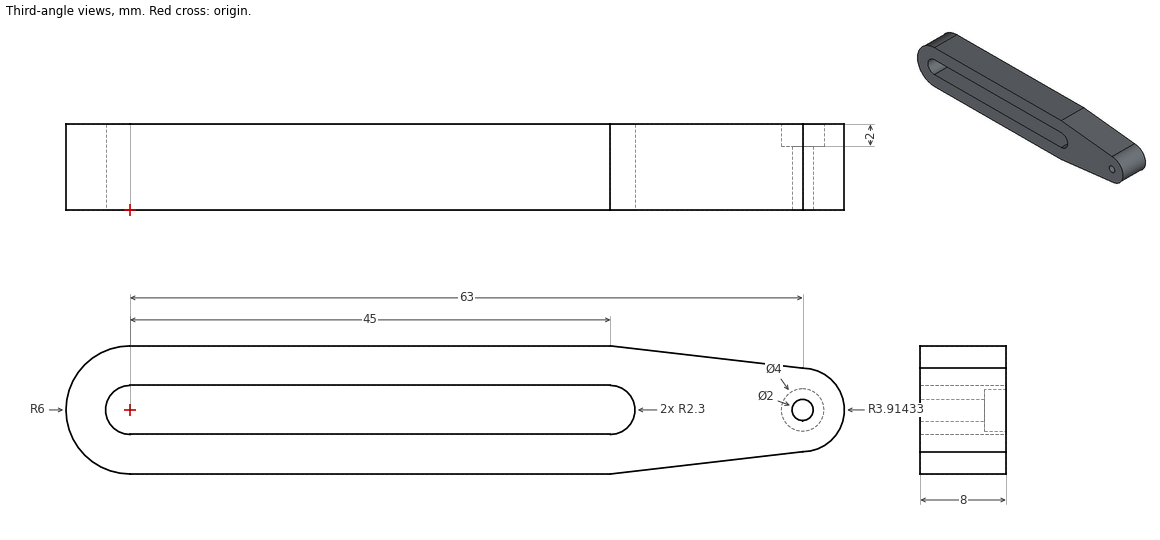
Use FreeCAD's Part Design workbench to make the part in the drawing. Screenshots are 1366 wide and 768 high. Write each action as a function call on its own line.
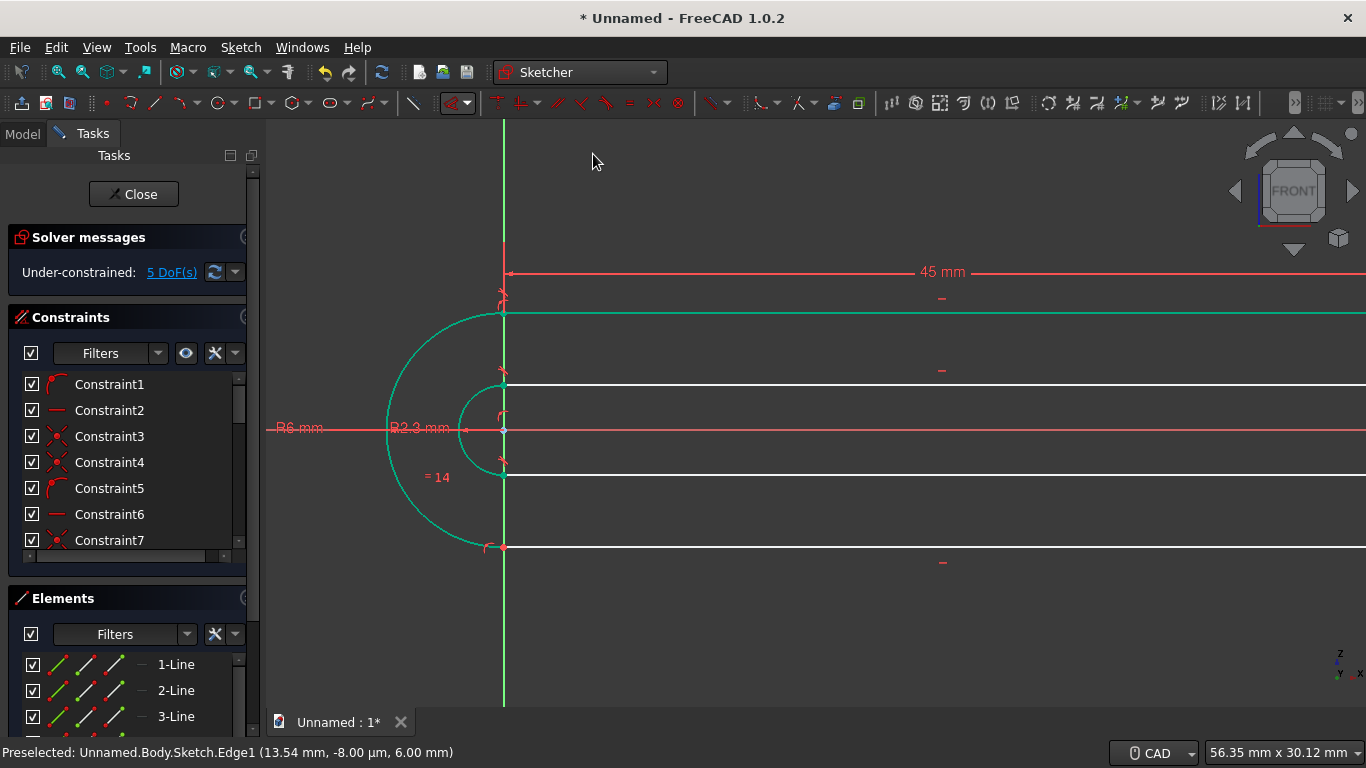
click(1119, 547)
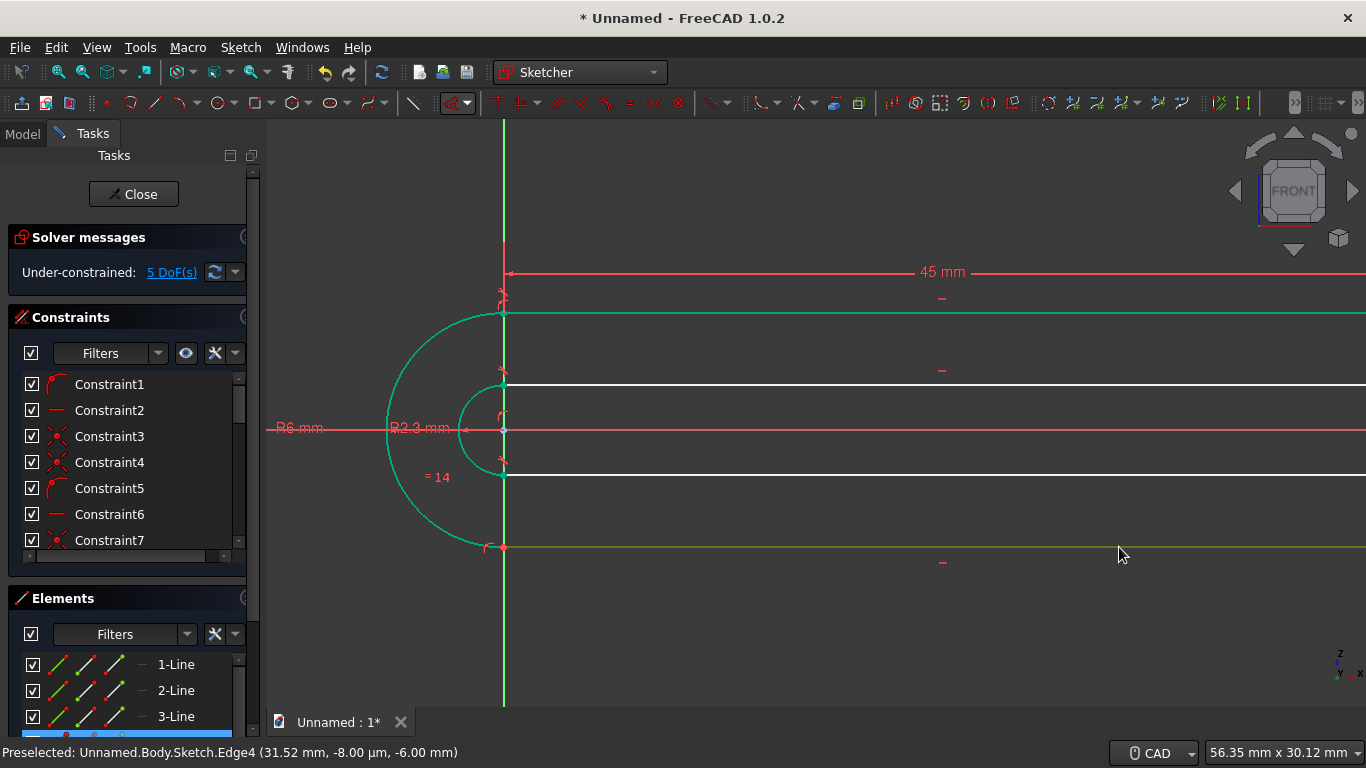
key(l)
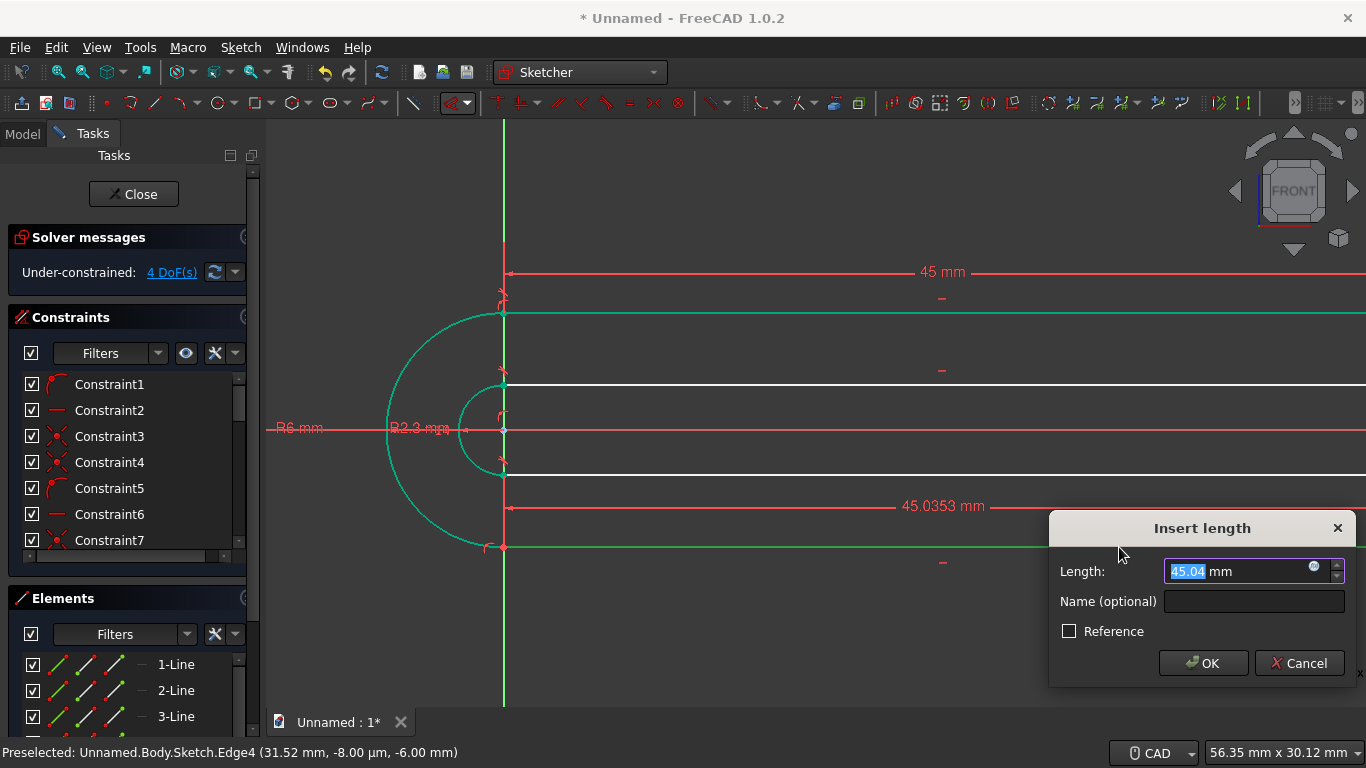
text(45)
key(Return)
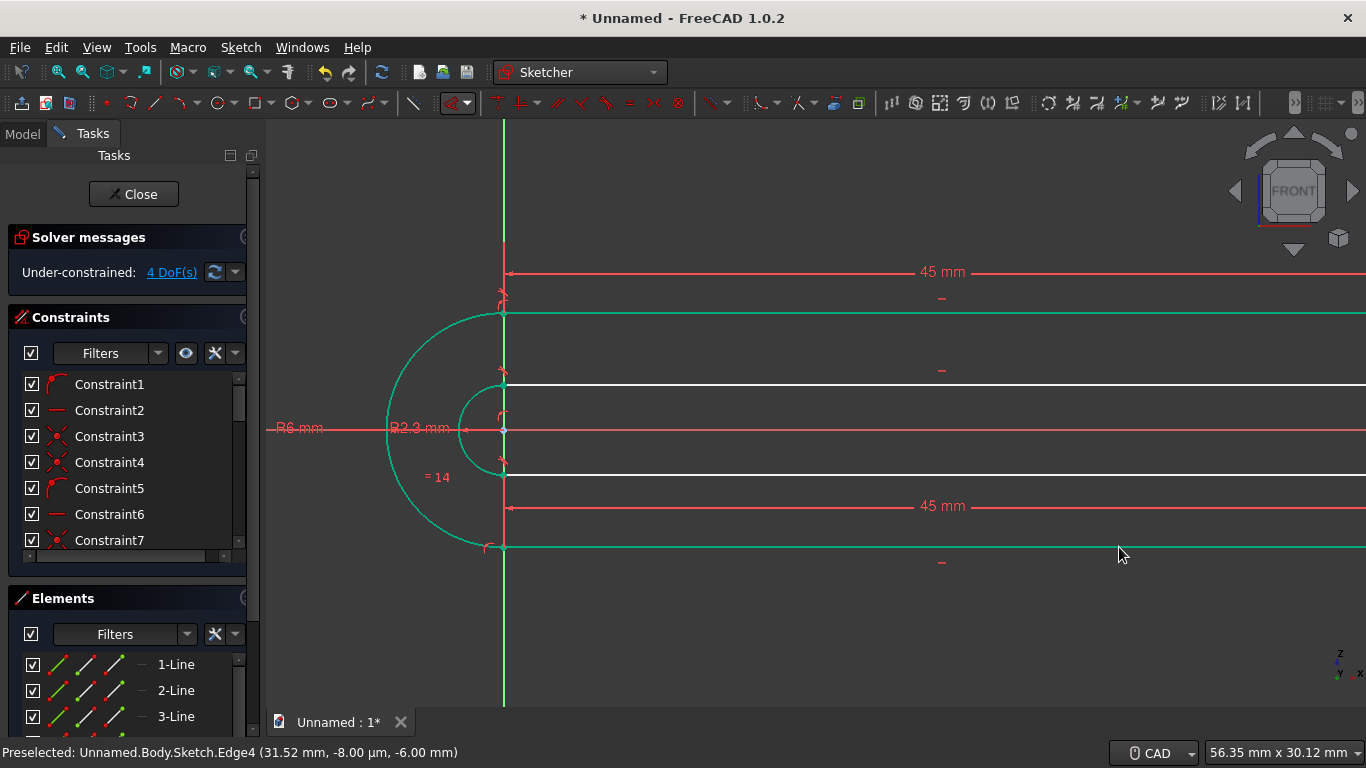
click(767, 385)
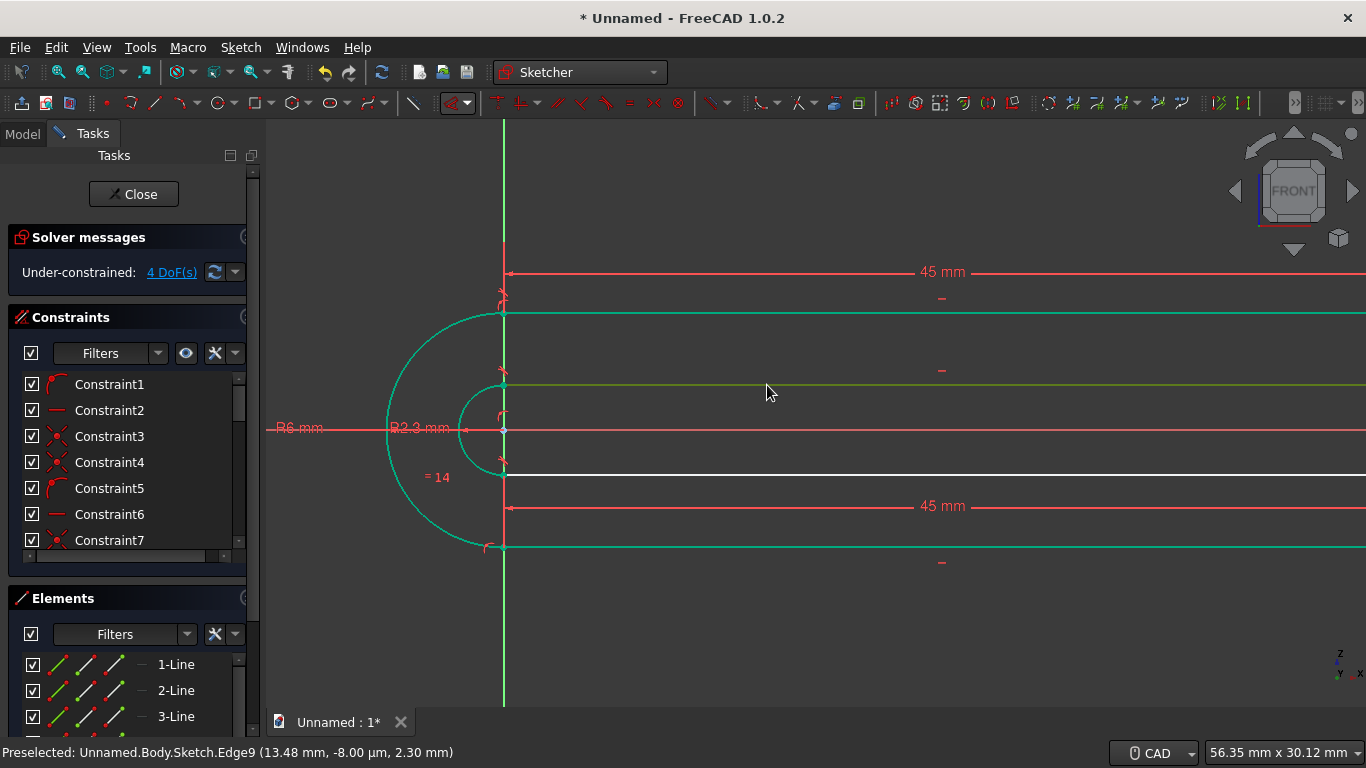
click(470, 104)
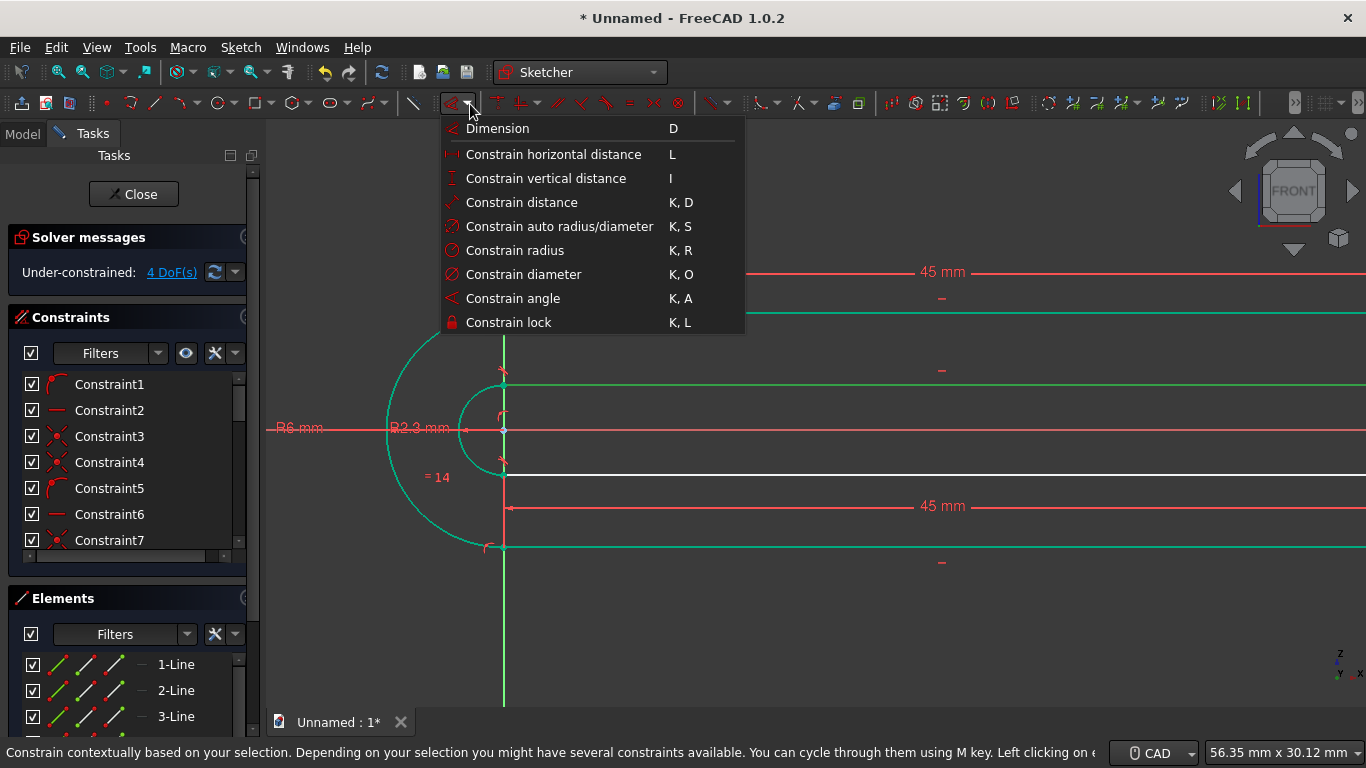
click(593, 154)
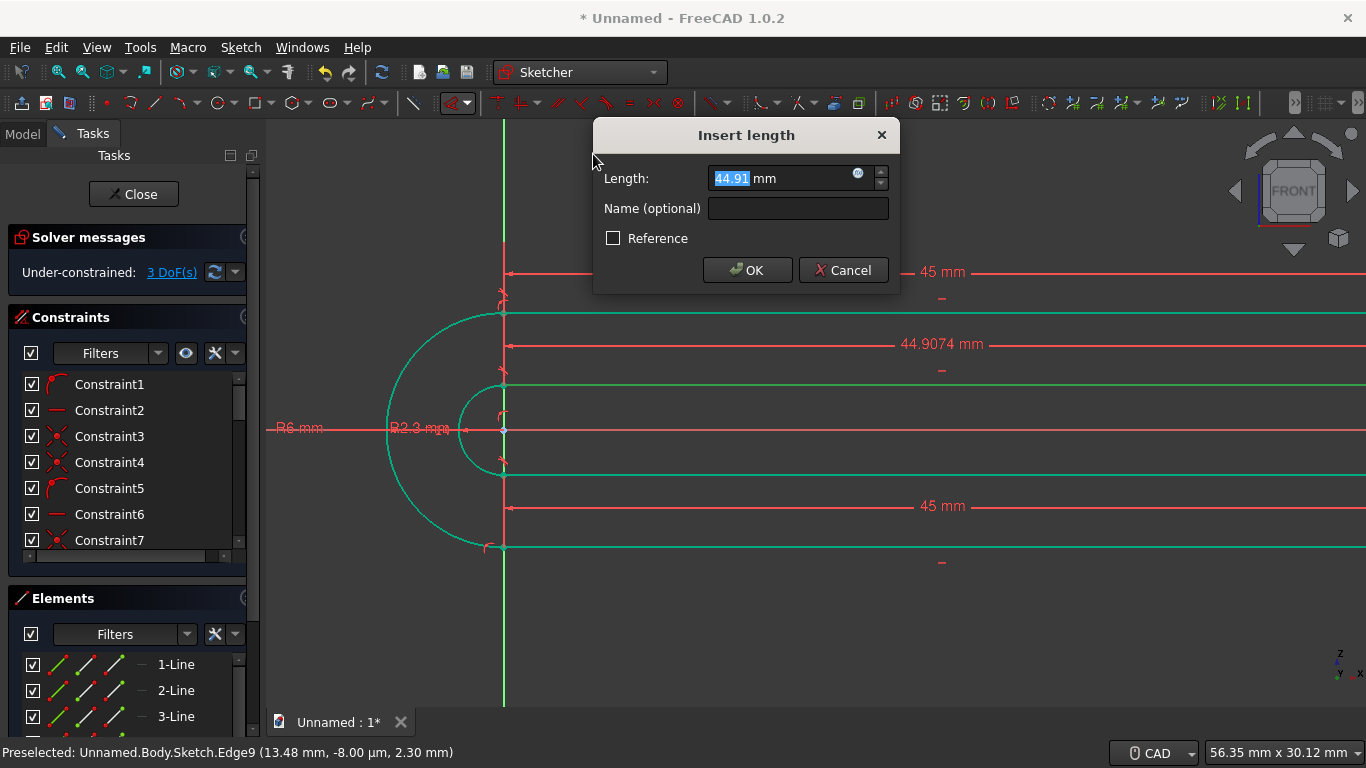
text(45)
key(Return)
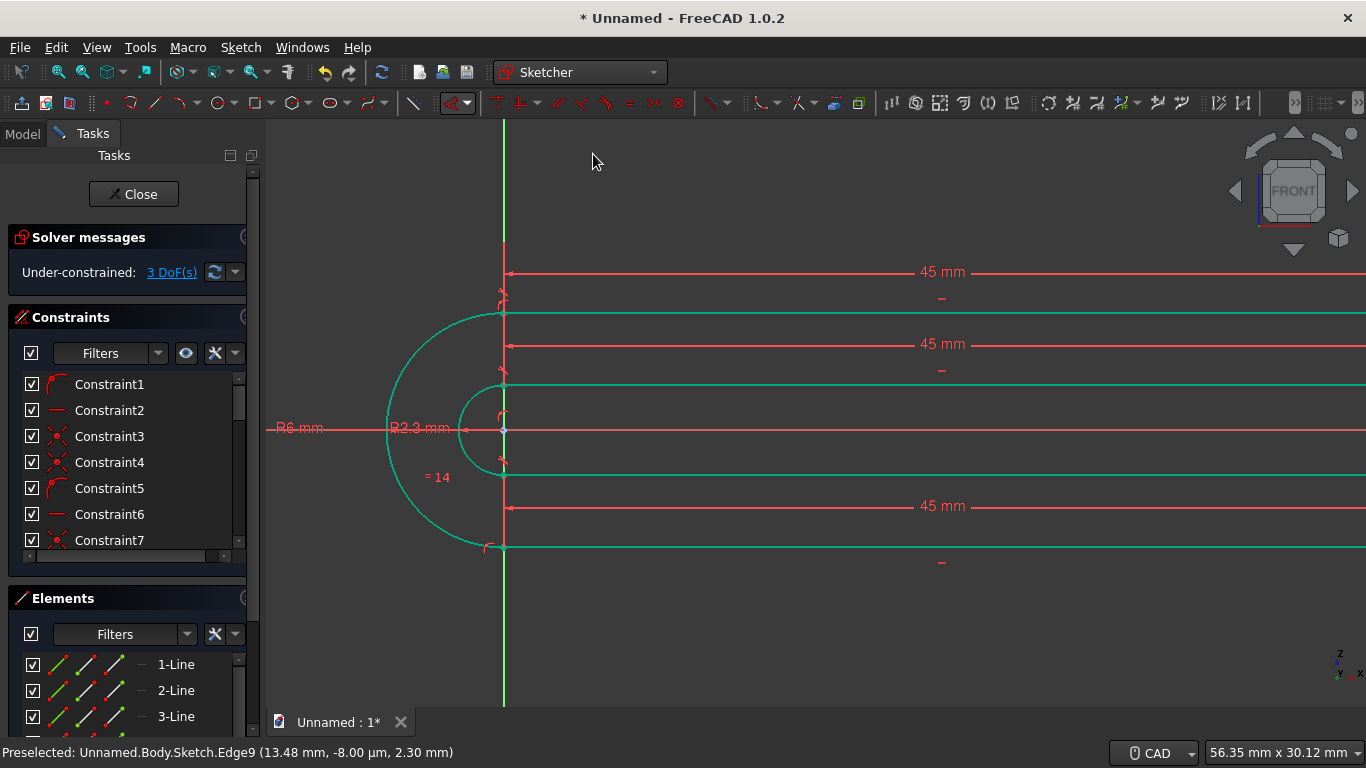
scroll(461, 399, down, 4)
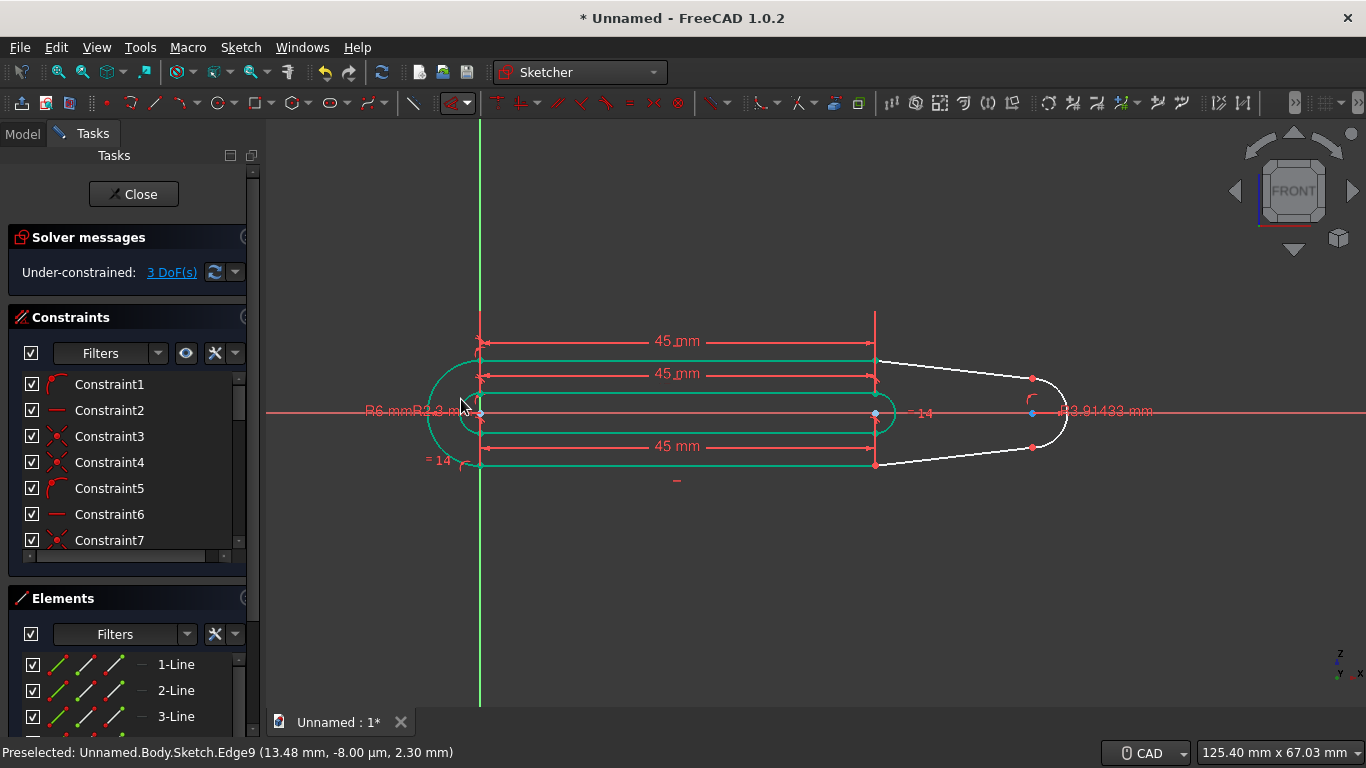
click(1033, 379)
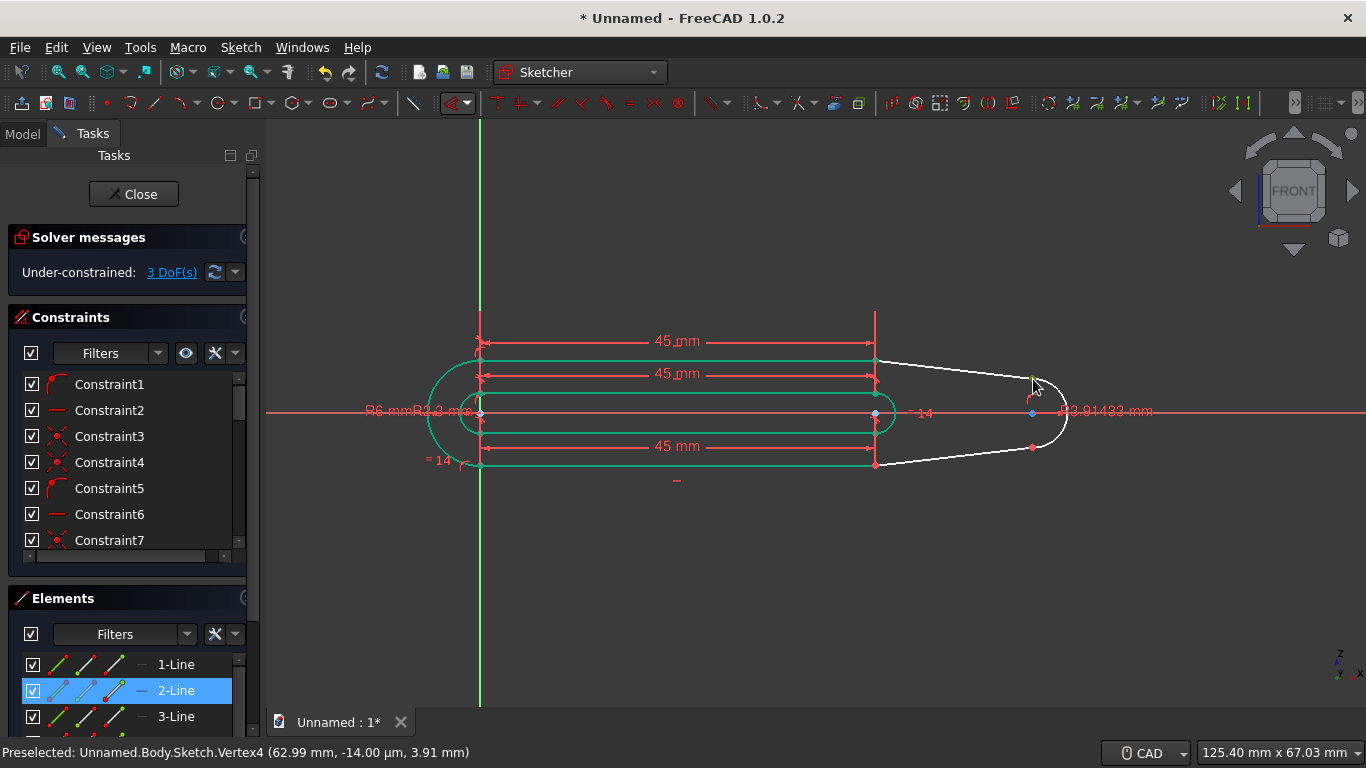
click(470, 104)